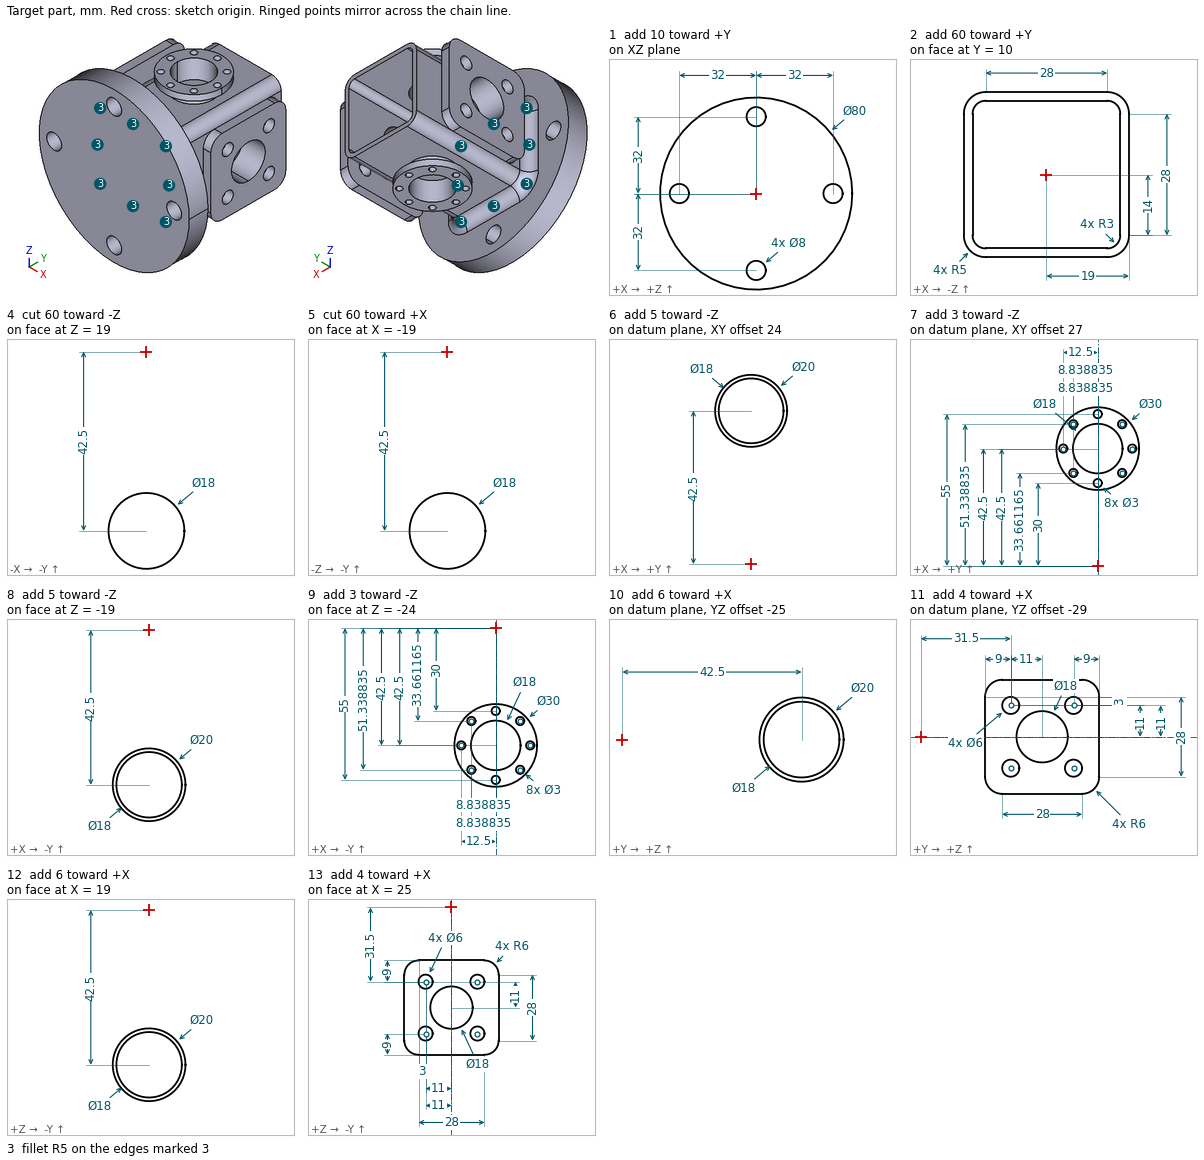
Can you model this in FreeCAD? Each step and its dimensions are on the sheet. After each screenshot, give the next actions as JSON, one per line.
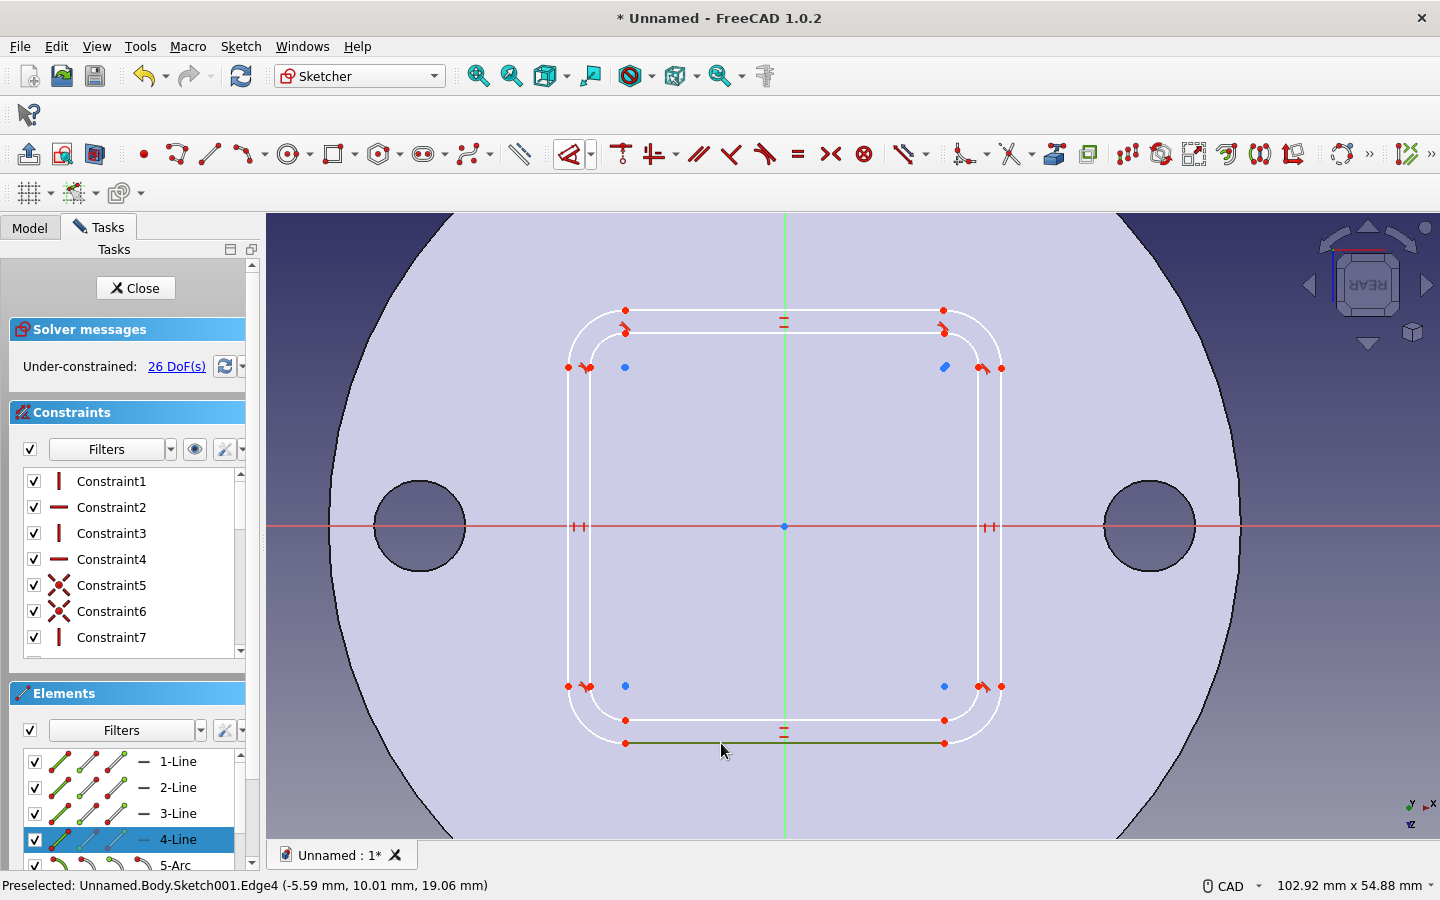
{"action": "left_click", "coordinate": [575, 712]}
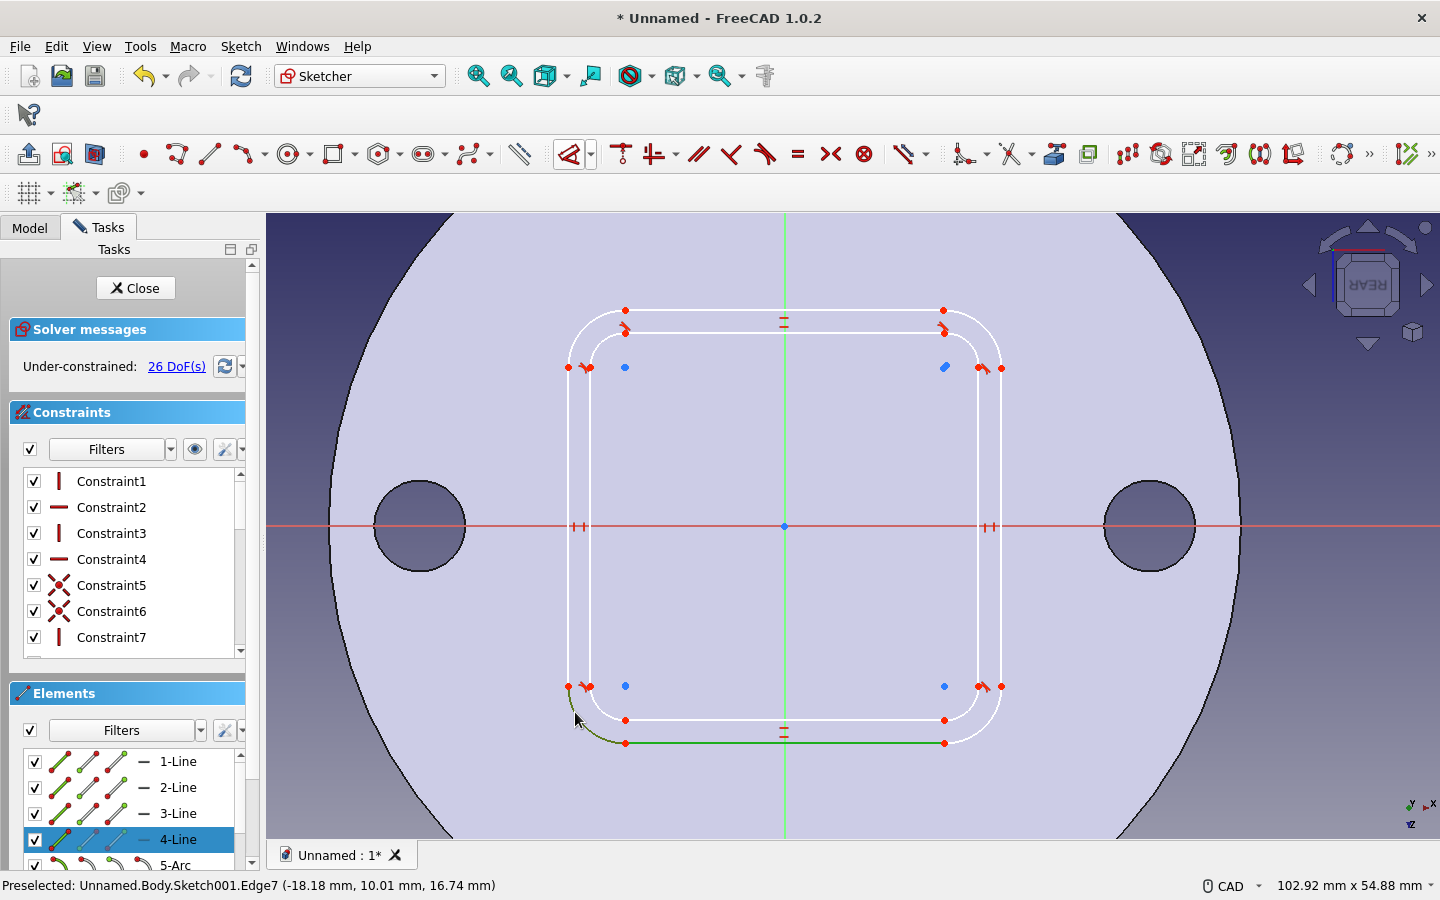
{"action": "key", "text": "t"}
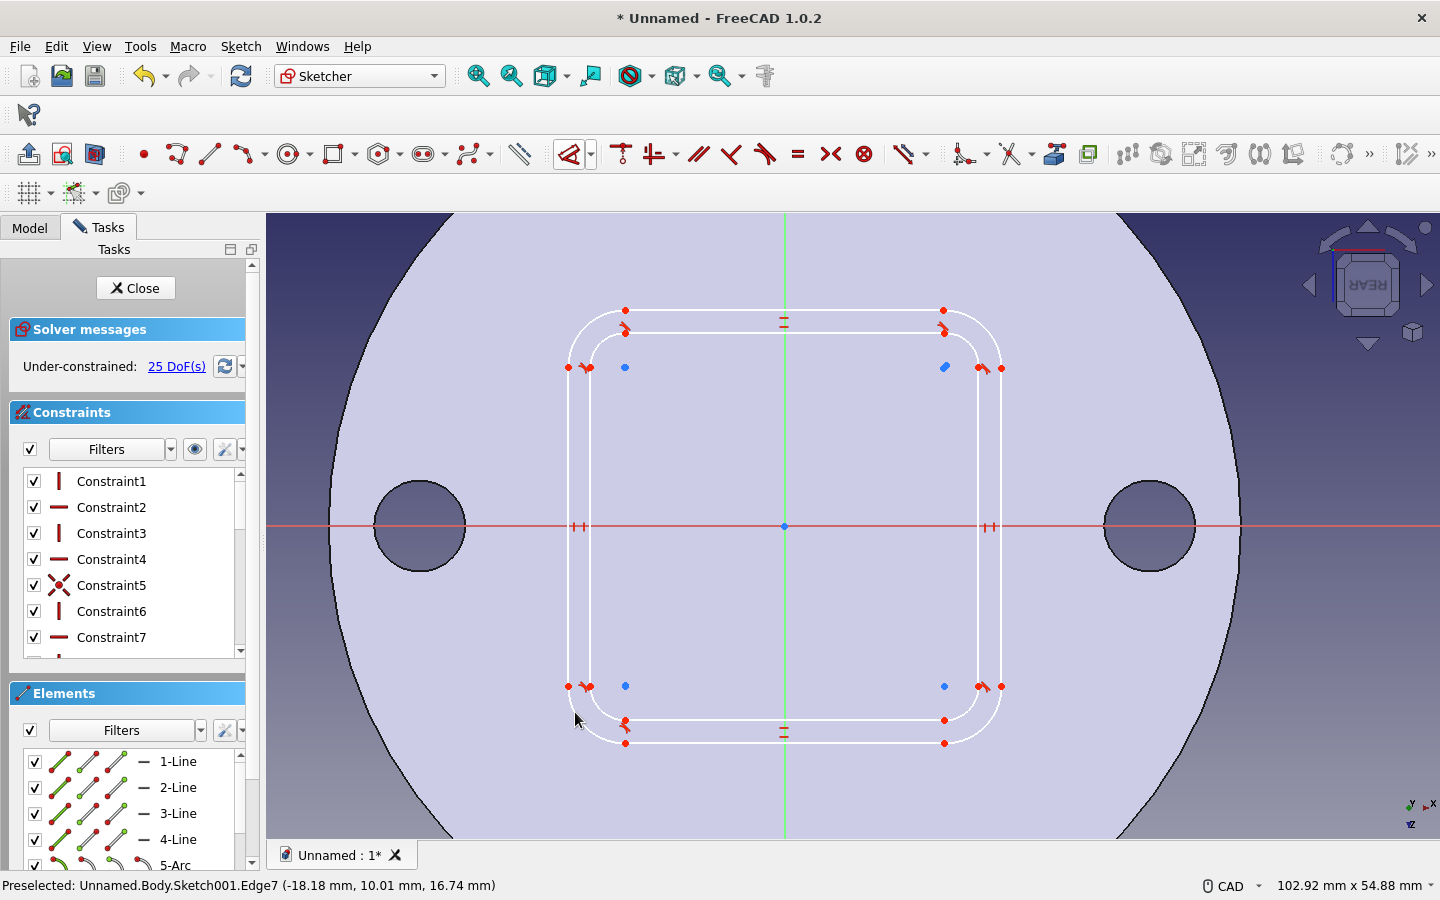
{"action": "left_click", "coordinate": [721, 743]}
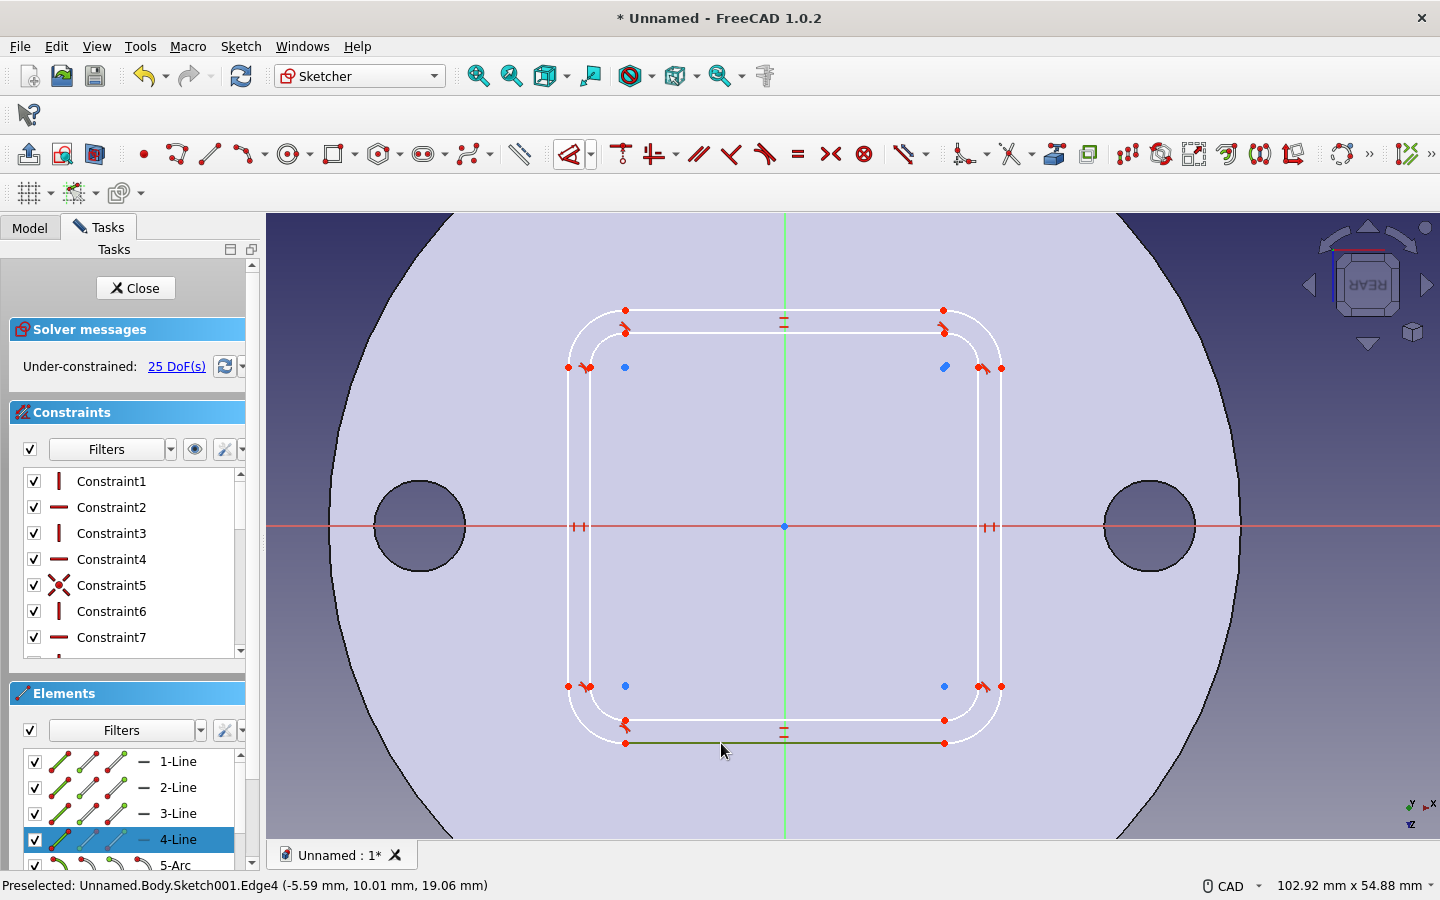
{"action": "left_click", "coordinate": [970, 737]}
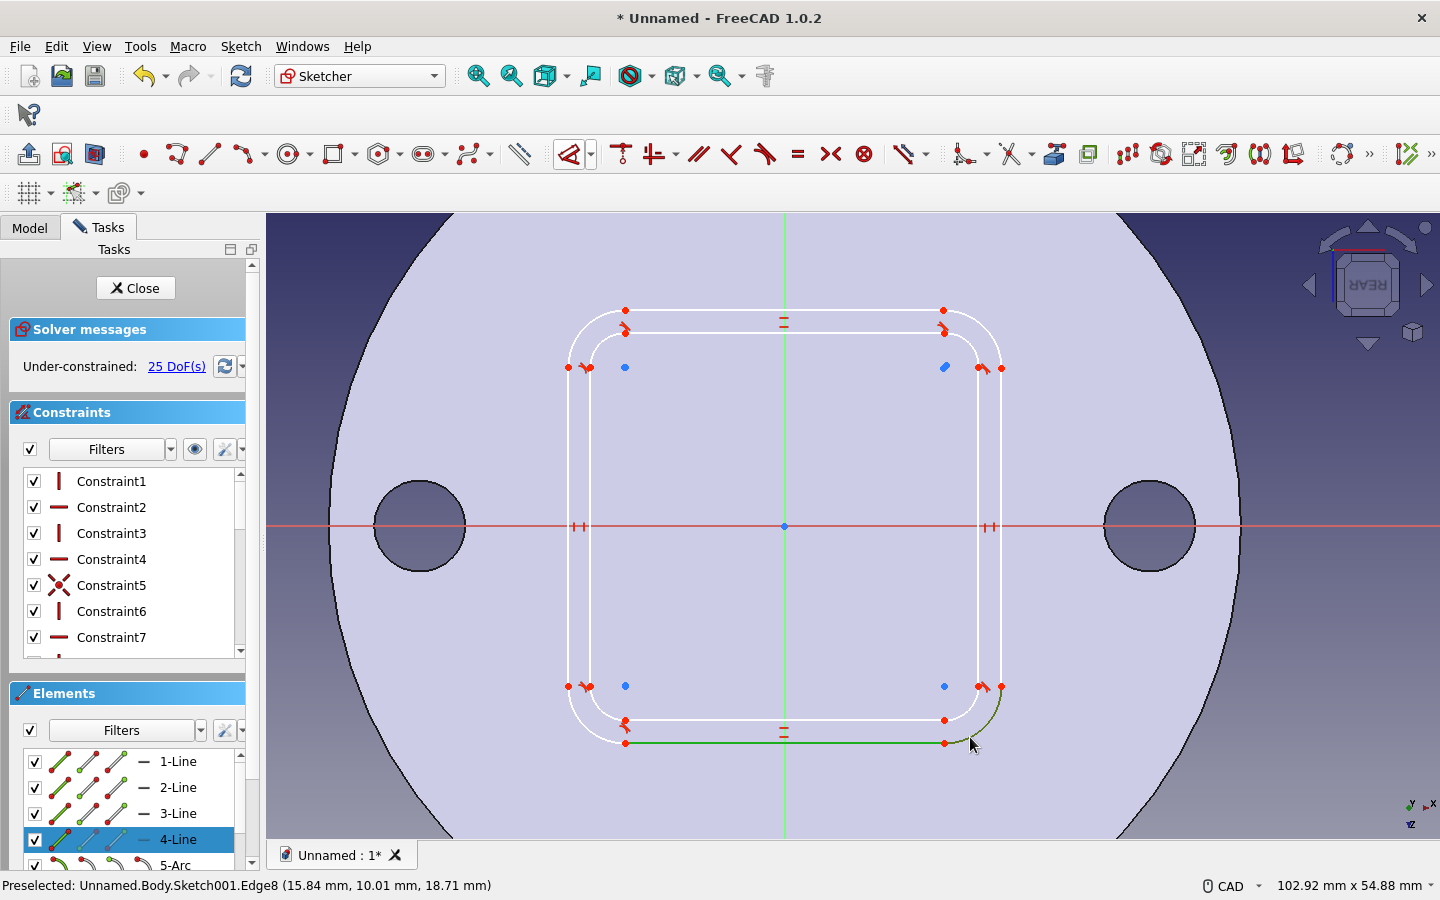
{"action": "key", "text": "t"}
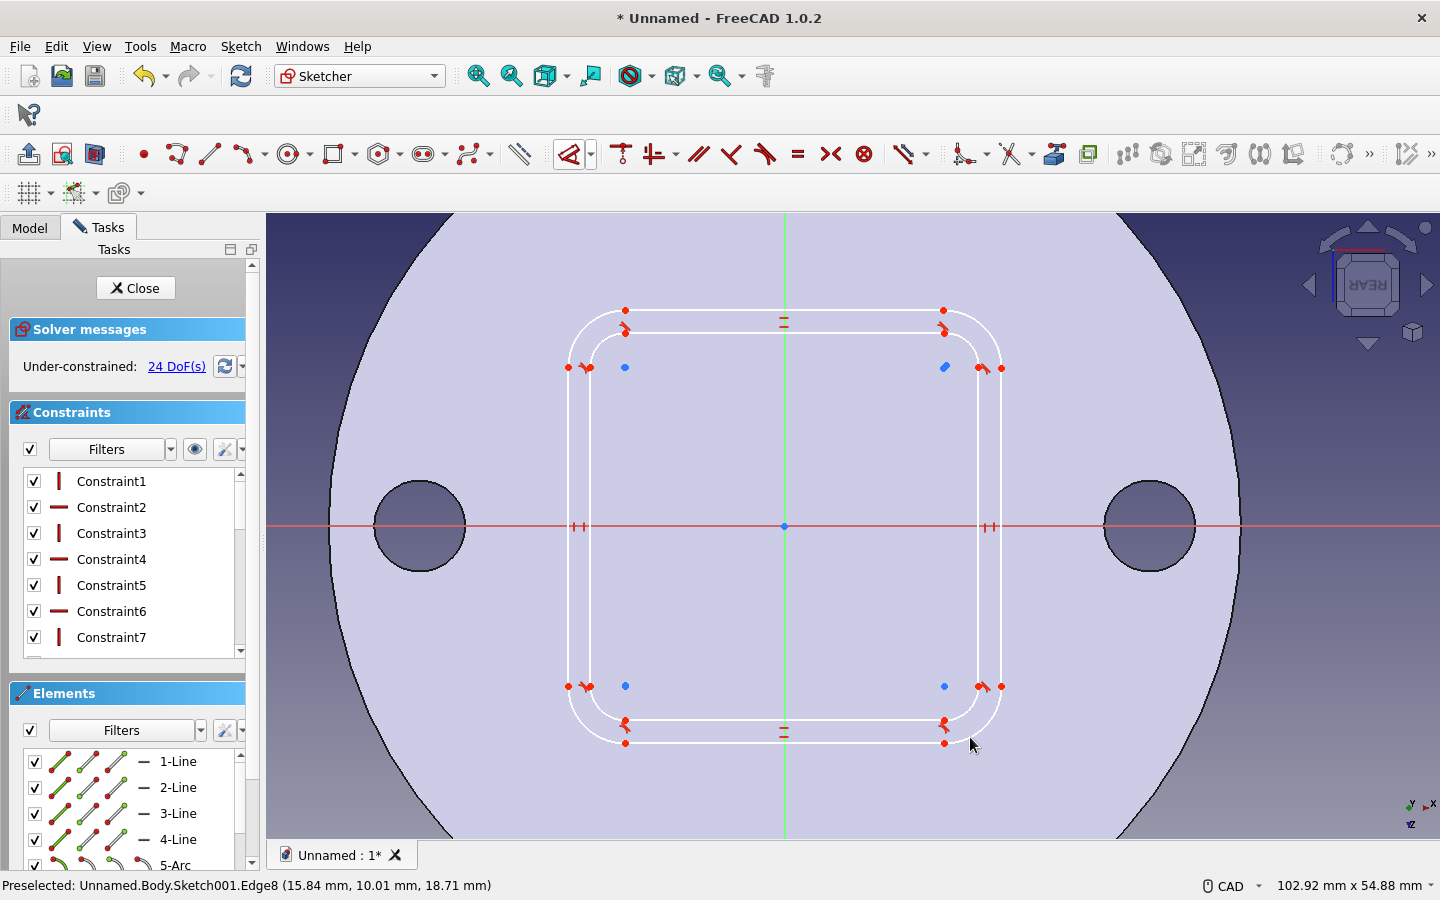
{"action": "left_click", "coordinate": [978, 463]}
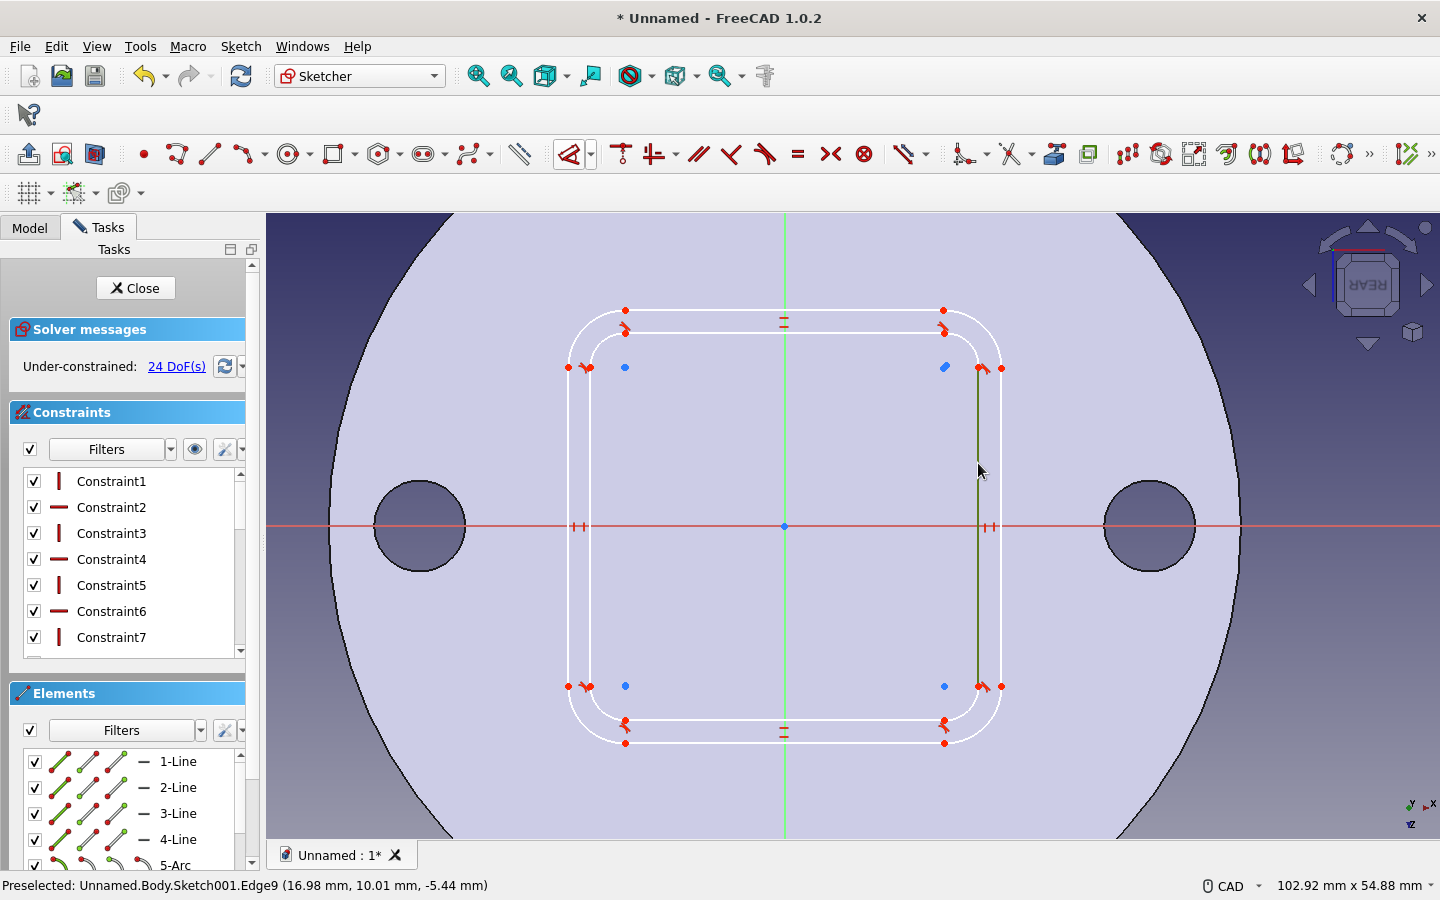
{"action": "left_click", "coordinate": [960, 717]}